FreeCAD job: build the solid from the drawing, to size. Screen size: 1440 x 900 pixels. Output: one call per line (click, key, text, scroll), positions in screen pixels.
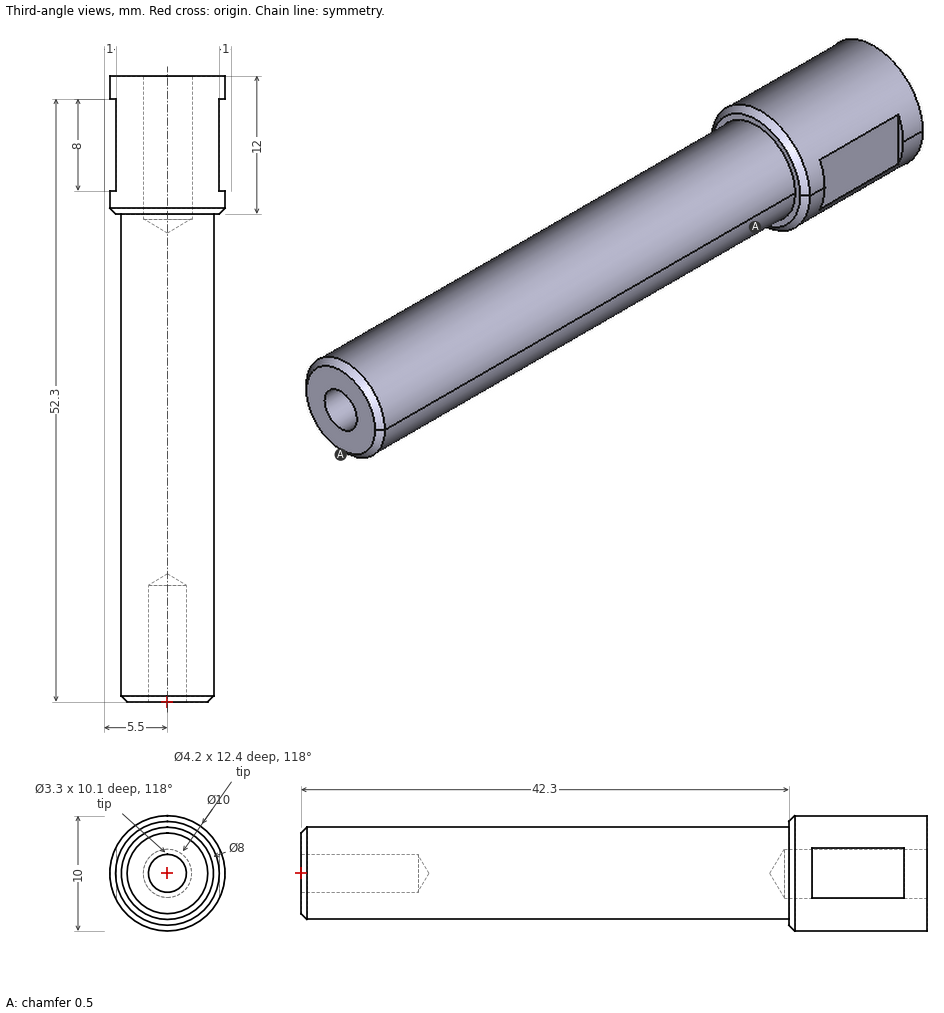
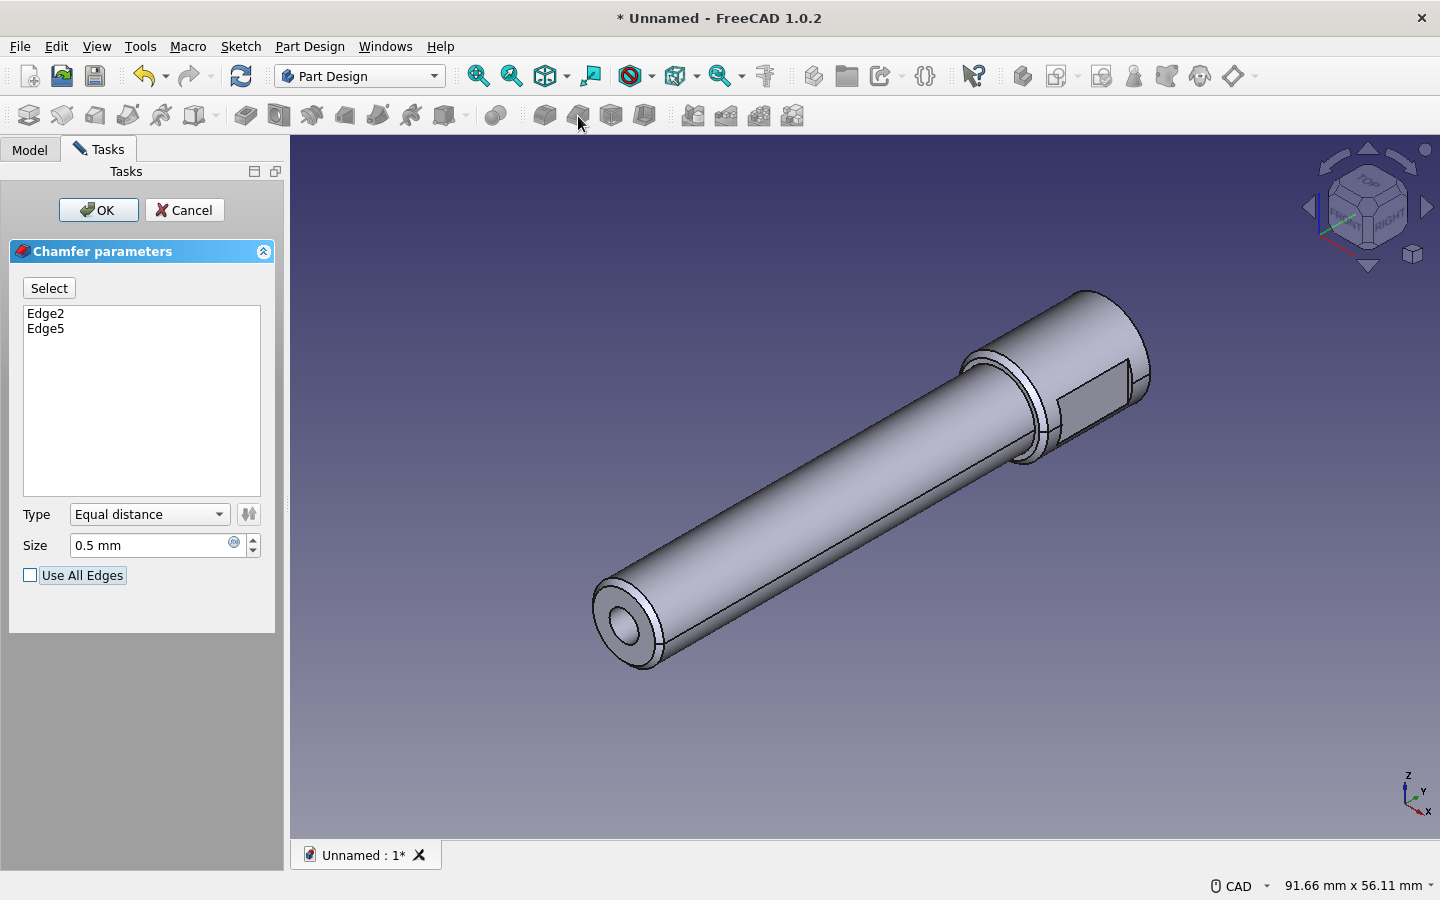
click(99, 210)